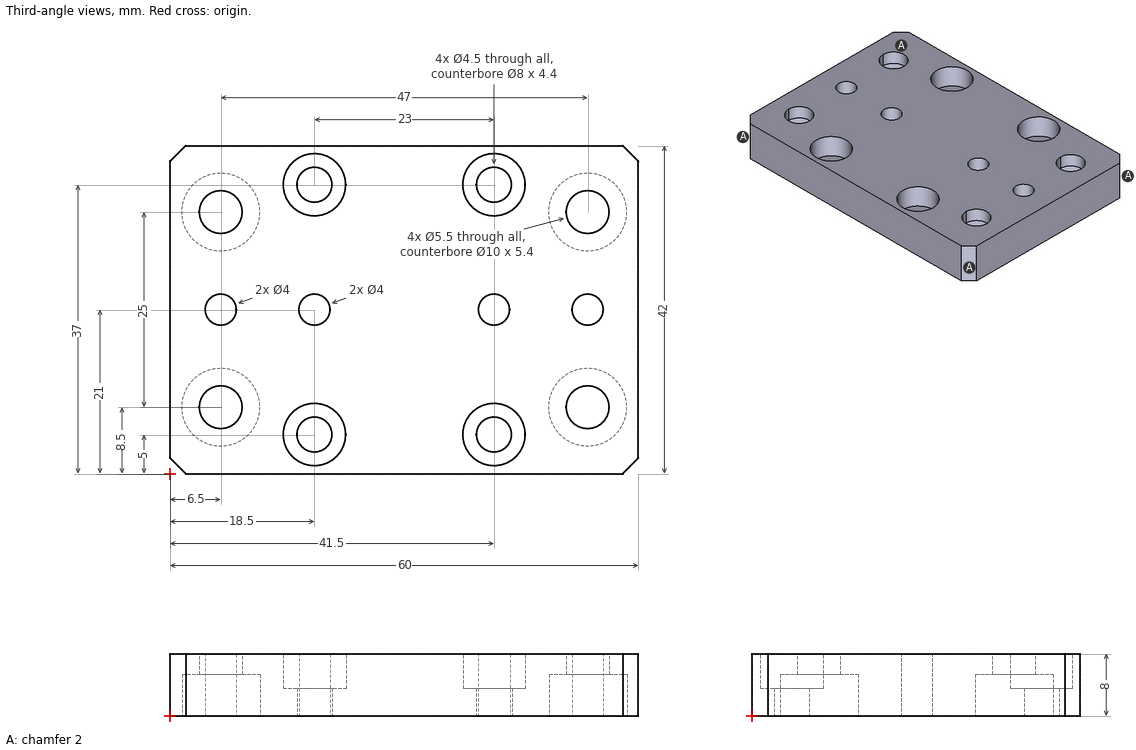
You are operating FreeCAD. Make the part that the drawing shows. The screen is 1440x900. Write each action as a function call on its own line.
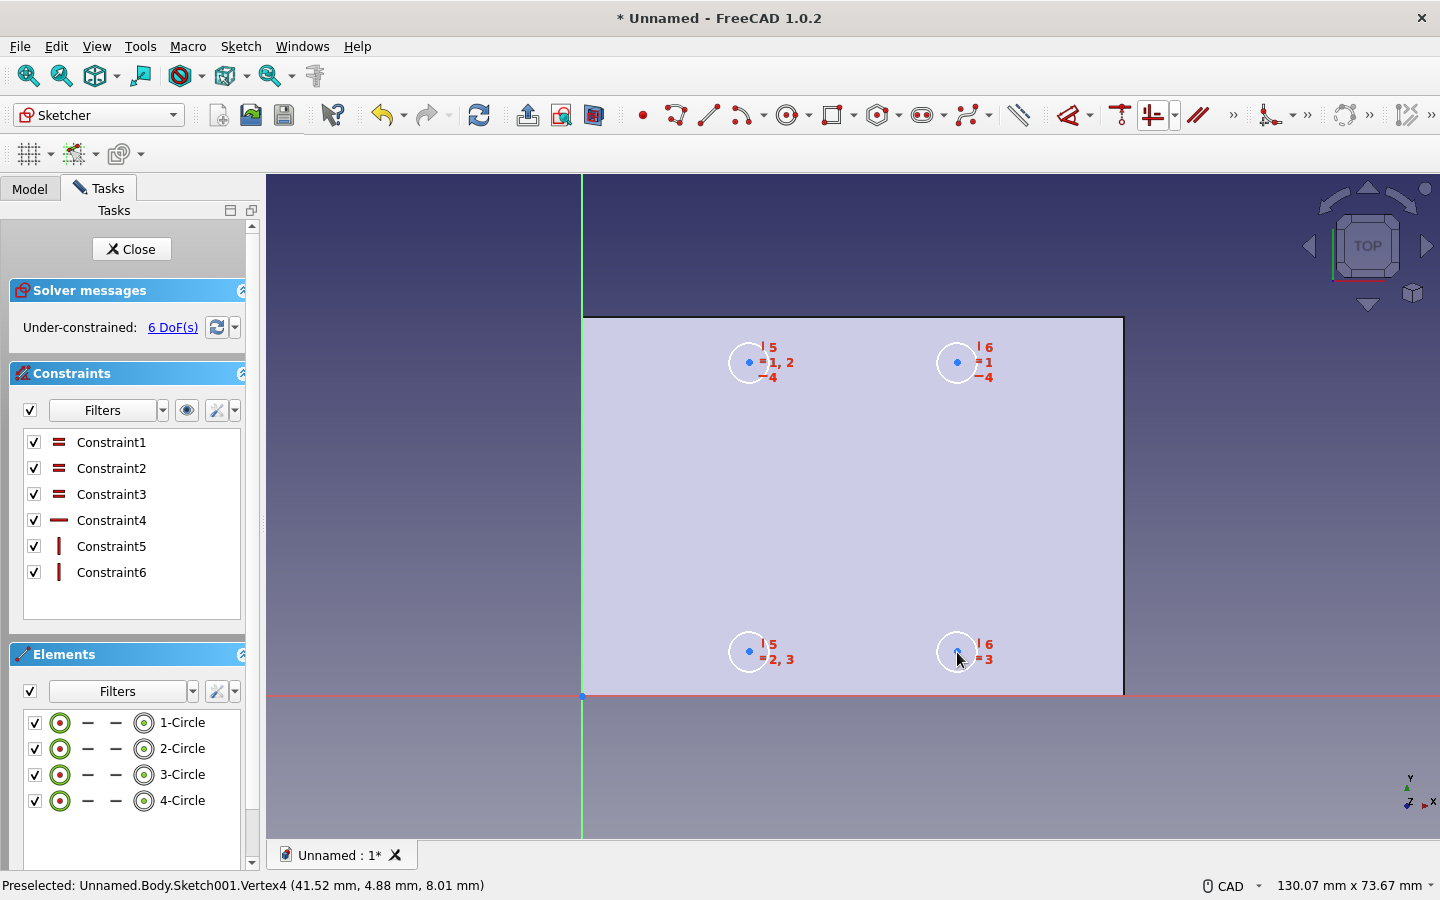
click(749, 652)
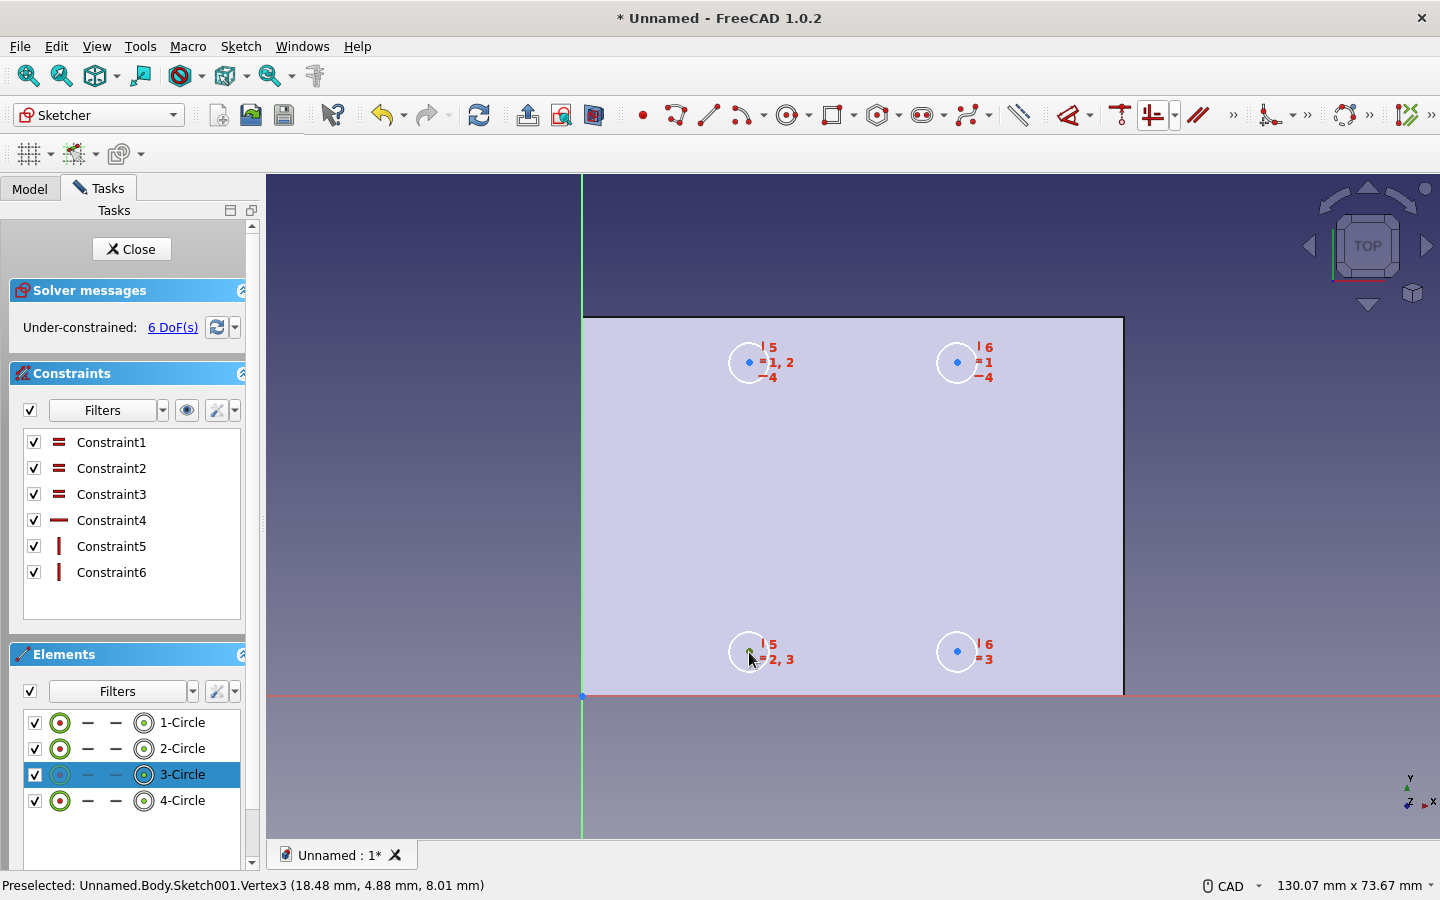
click(957, 652)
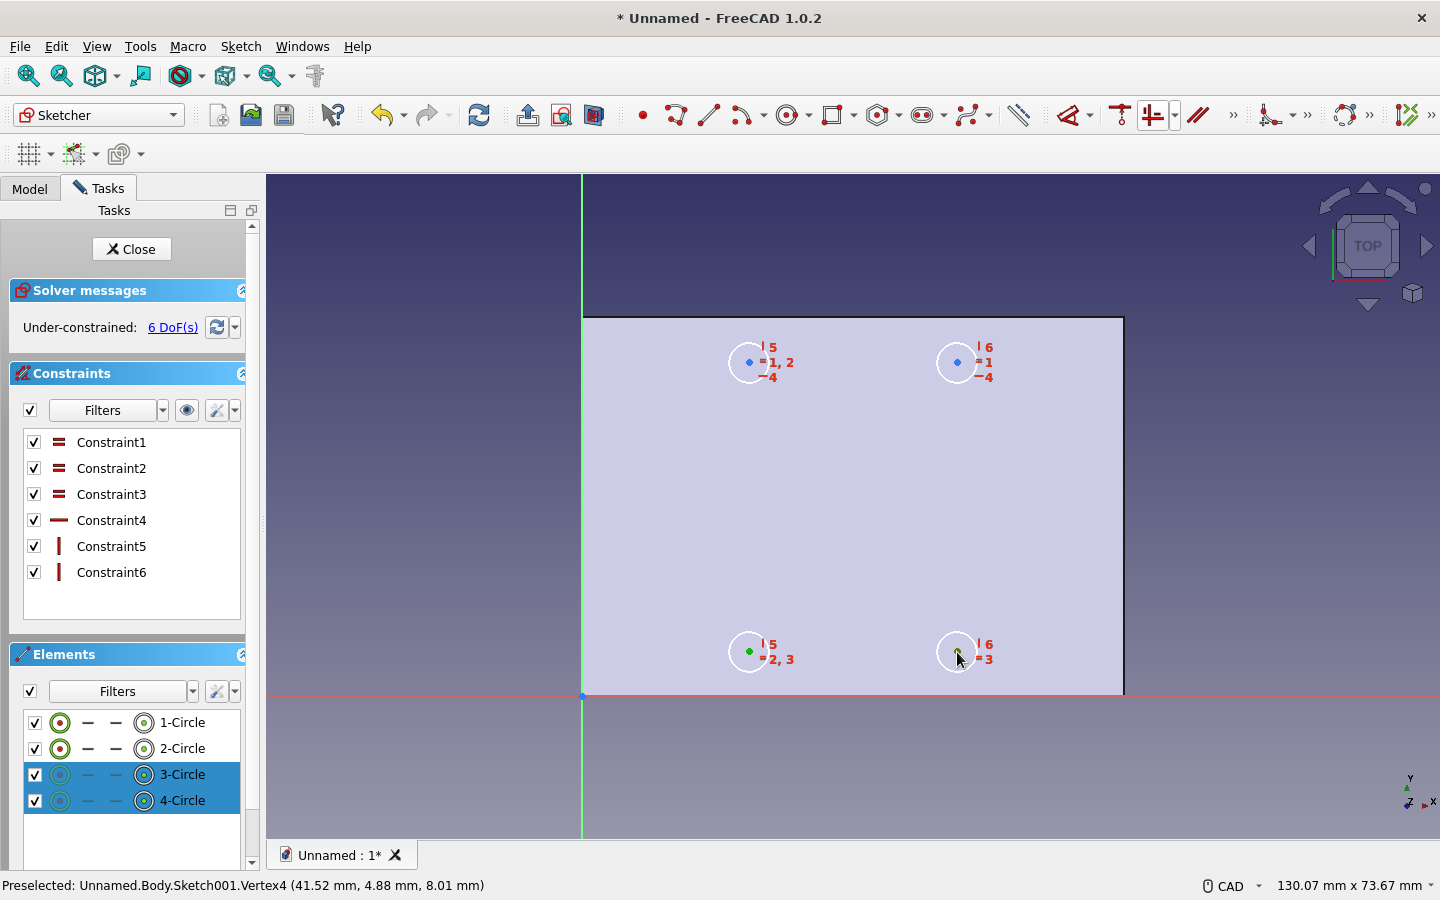
key(h)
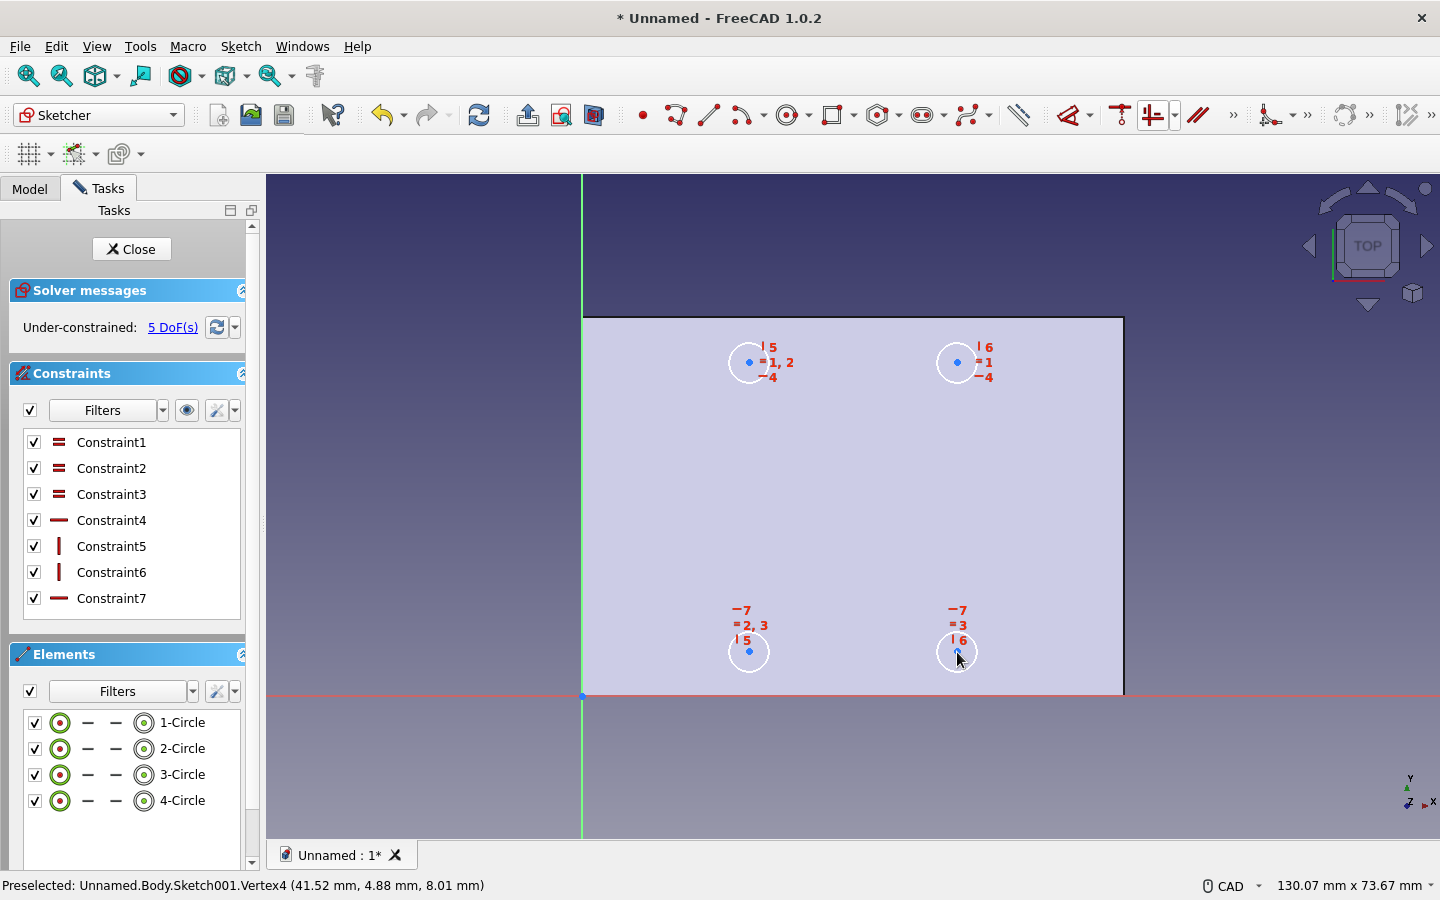
click(971, 349)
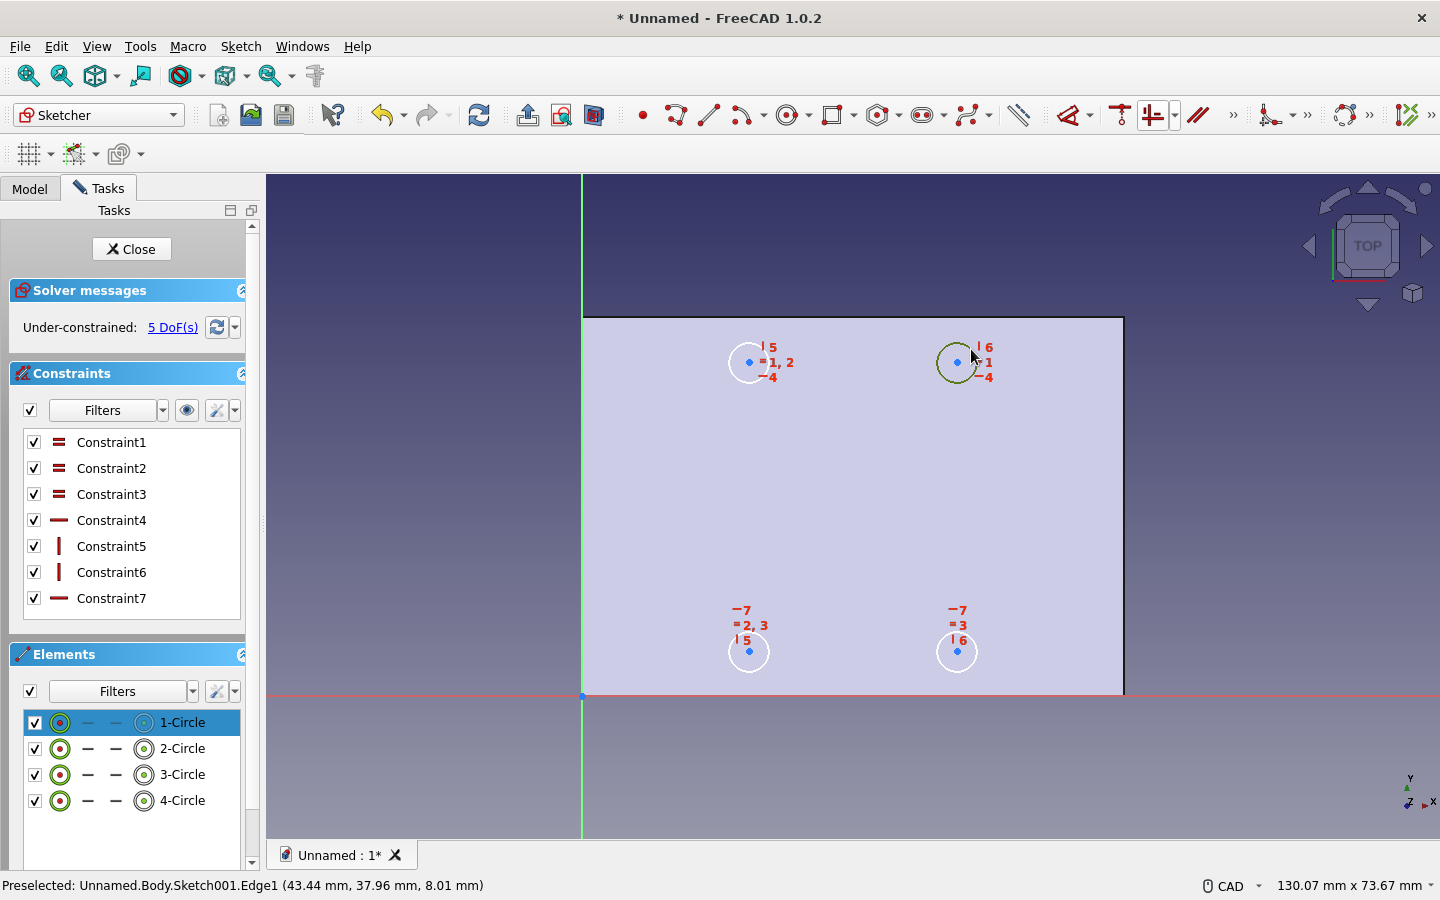
click(1090, 116)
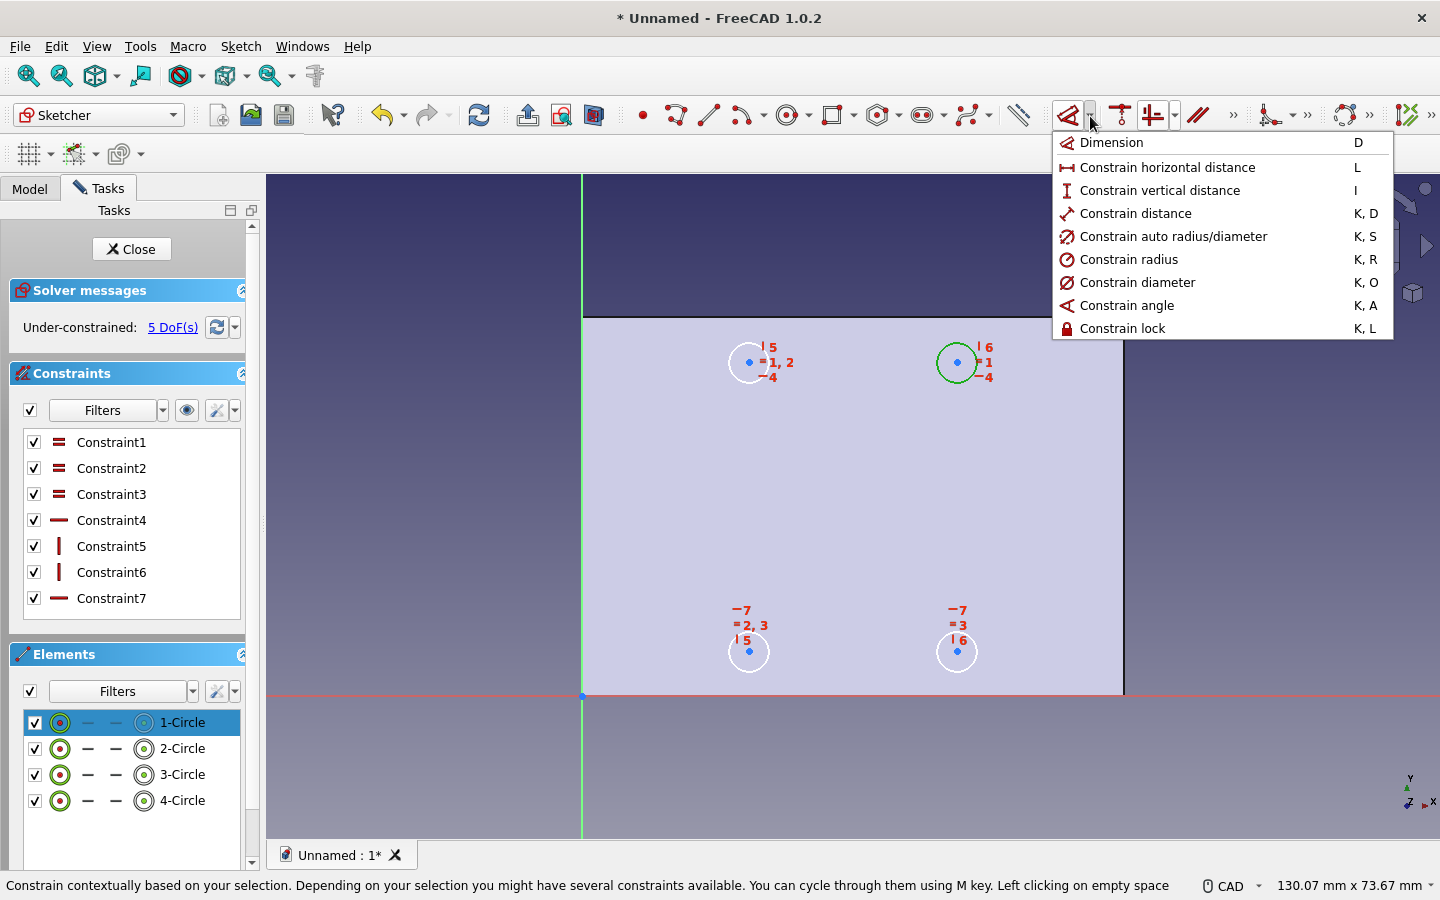
click(1223, 282)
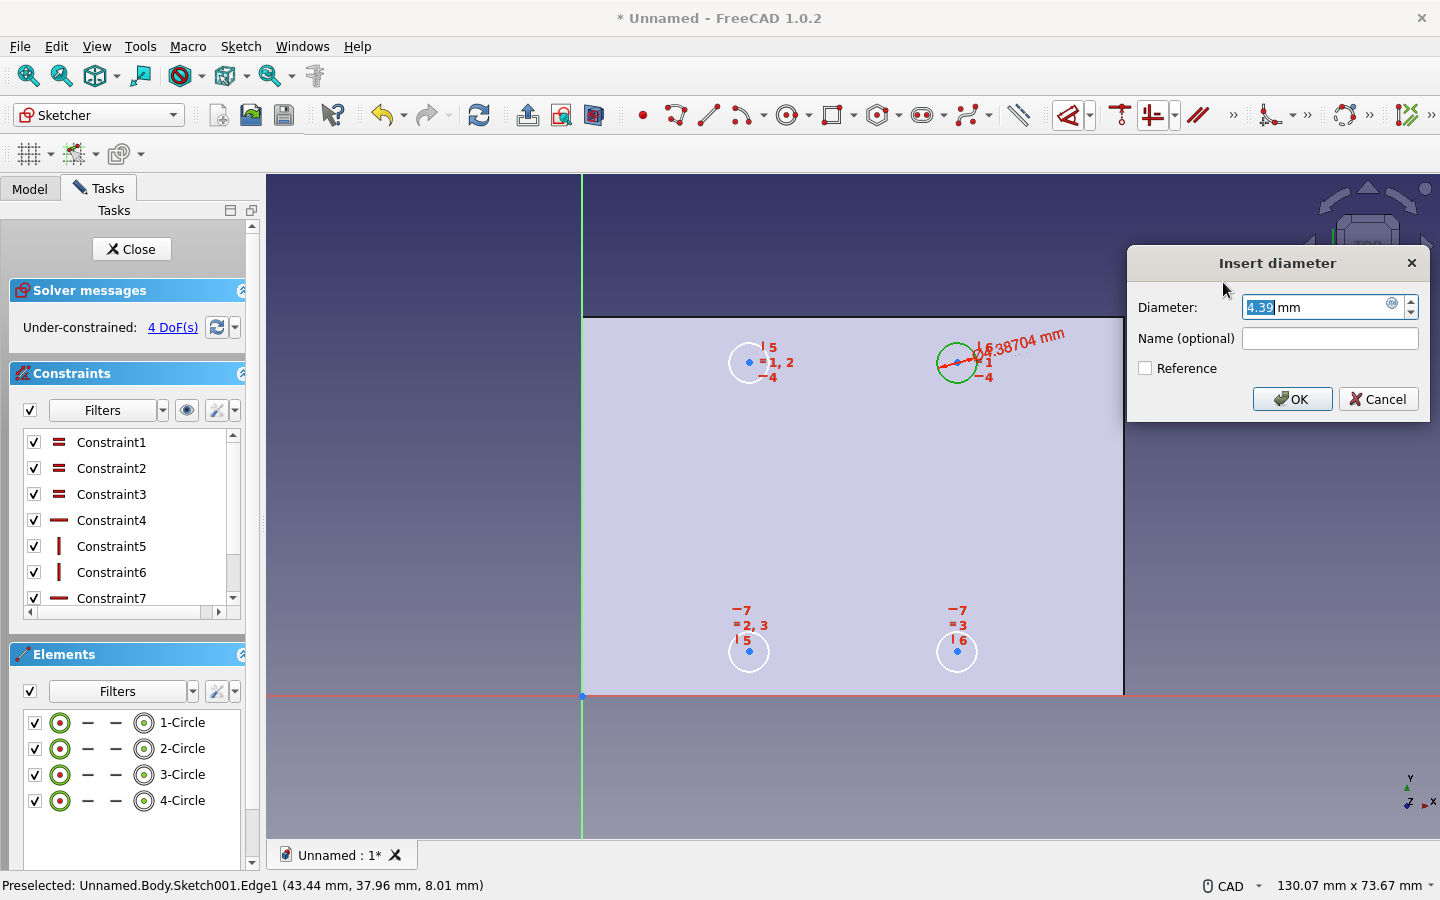
text(4.5)
key(Return)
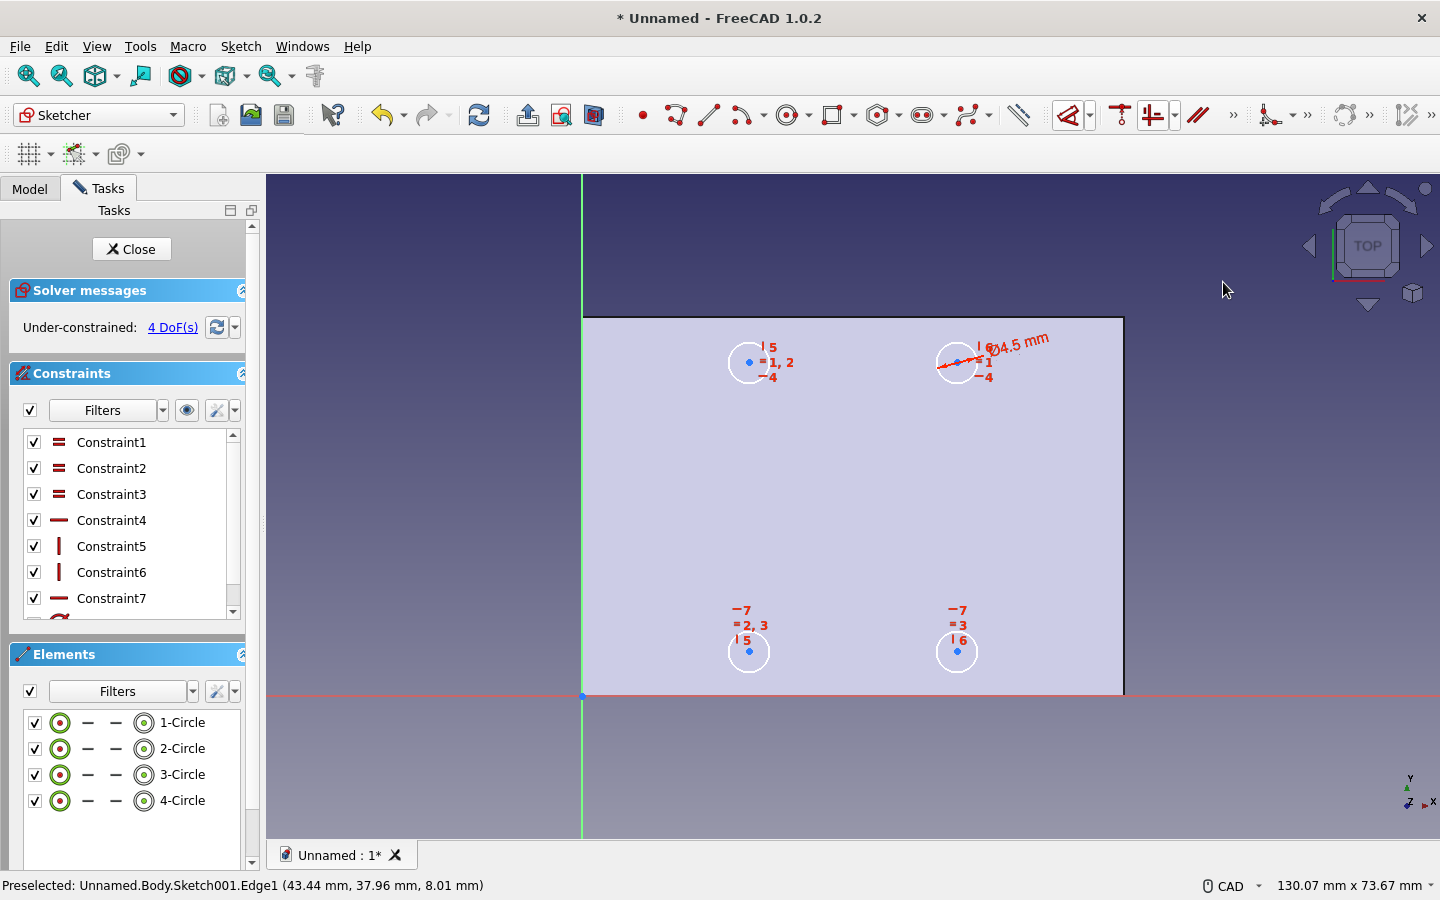
click(749, 652)